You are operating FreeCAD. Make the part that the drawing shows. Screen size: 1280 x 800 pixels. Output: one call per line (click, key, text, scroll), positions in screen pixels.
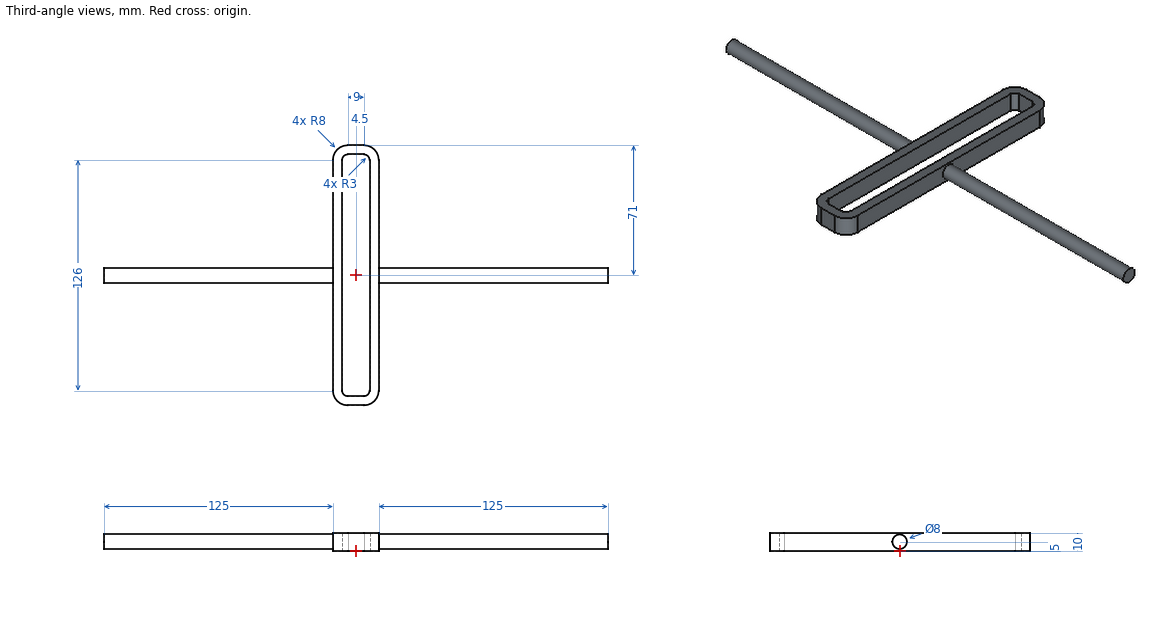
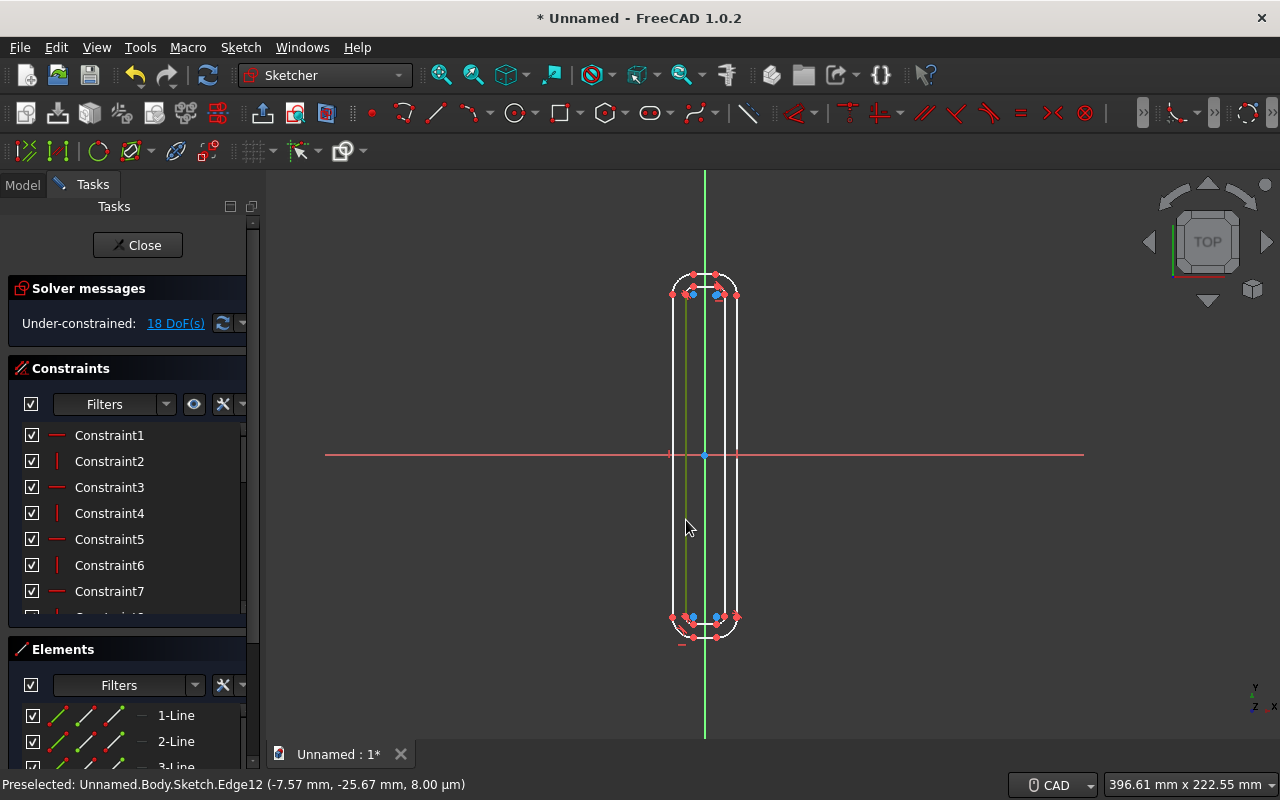
scroll(688, 622, up, 5)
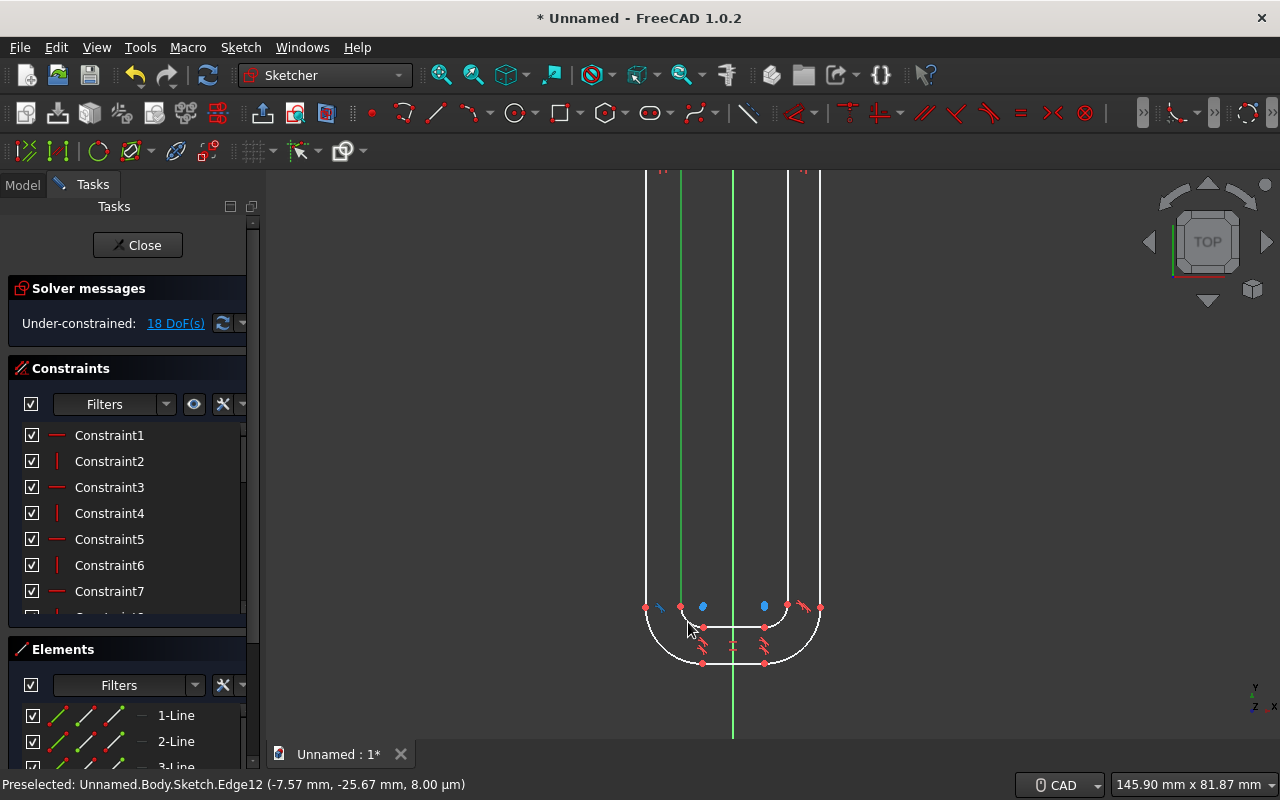
click(688, 621)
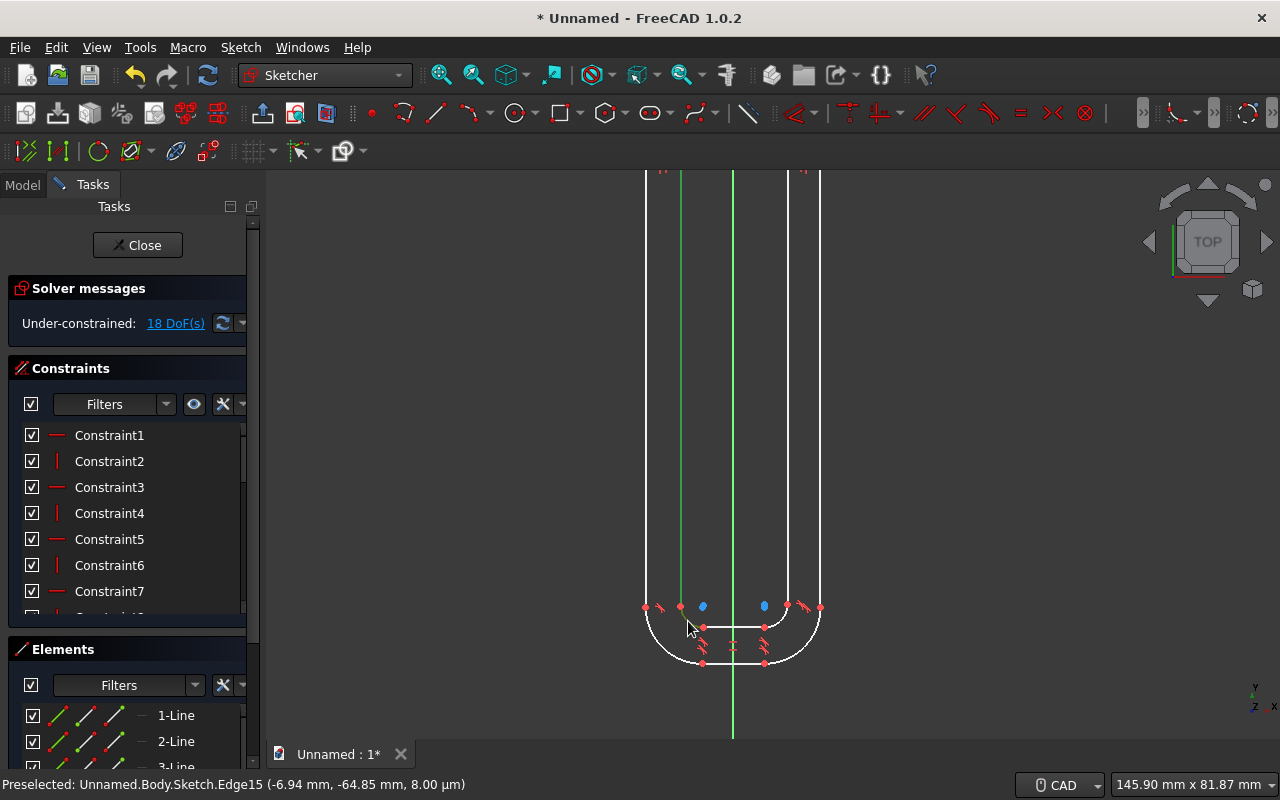
click(990, 114)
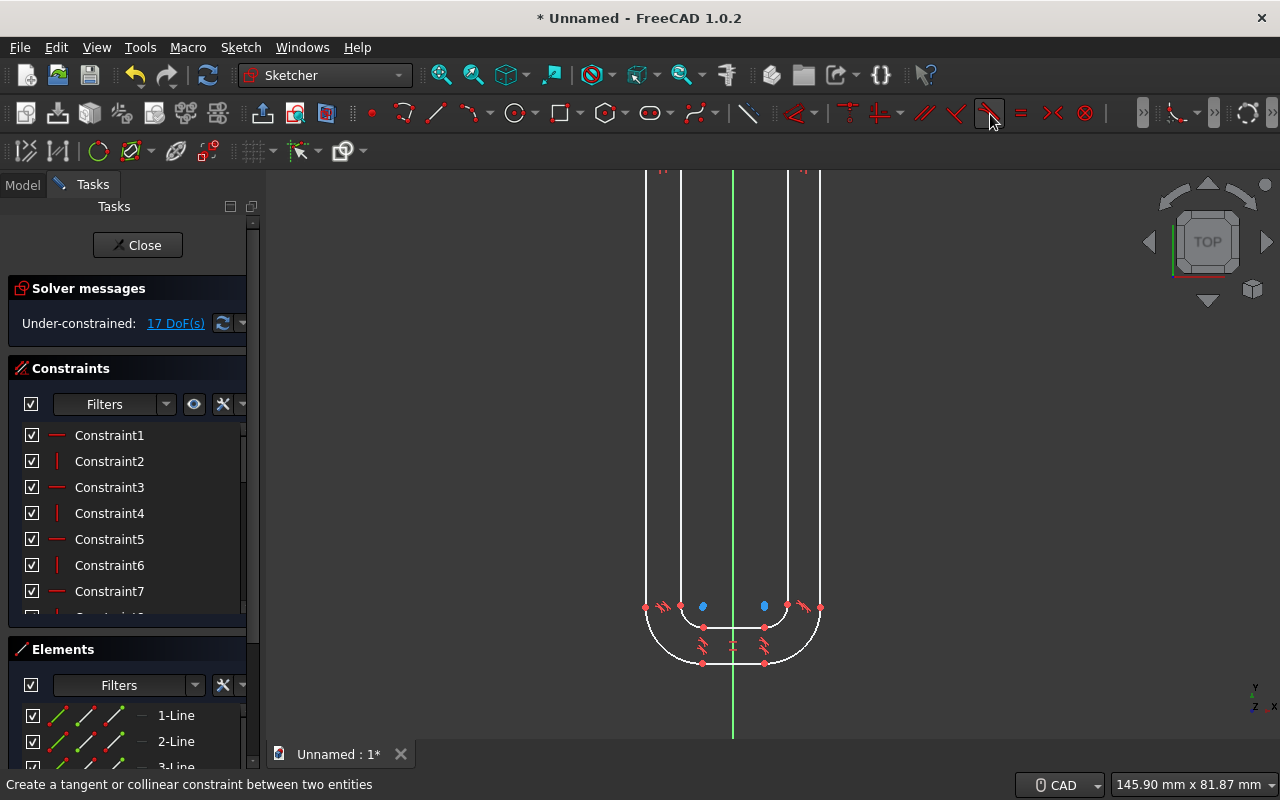
click(681, 343)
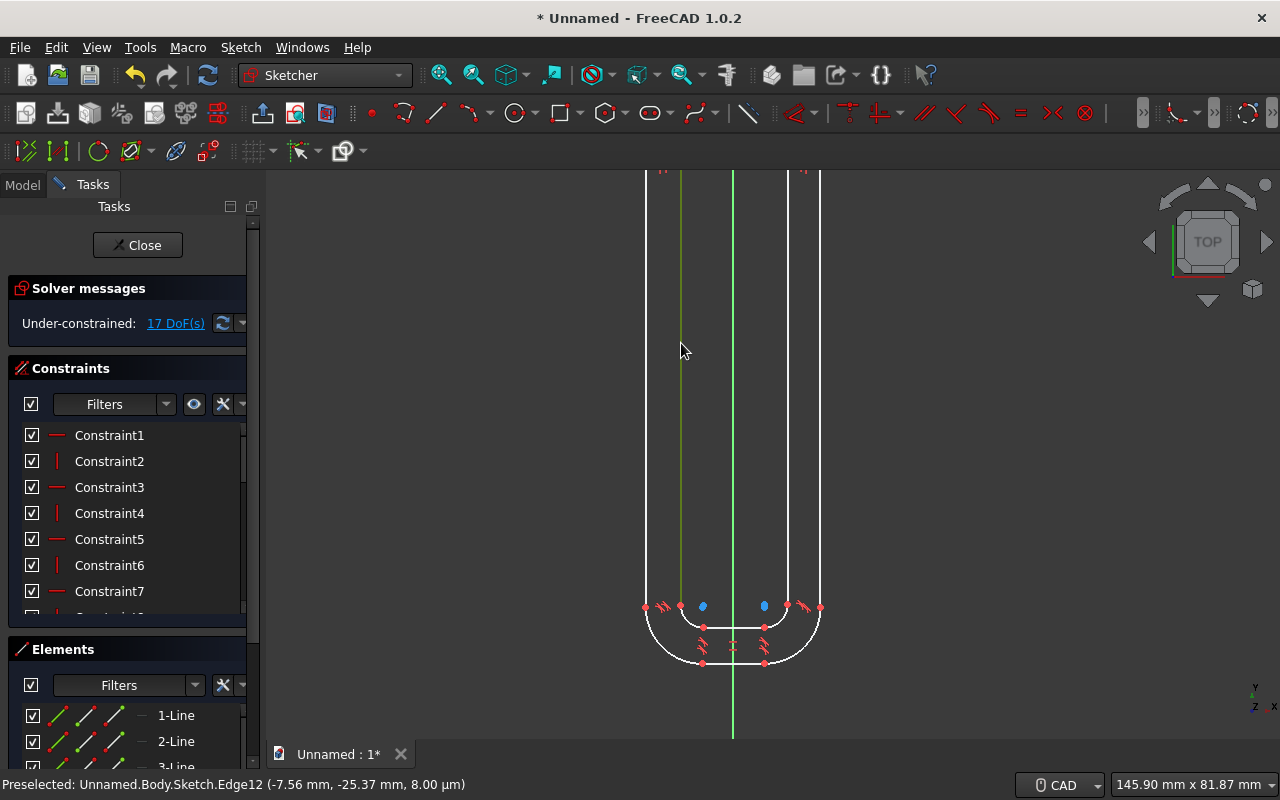
scroll(688, 621, down, 5)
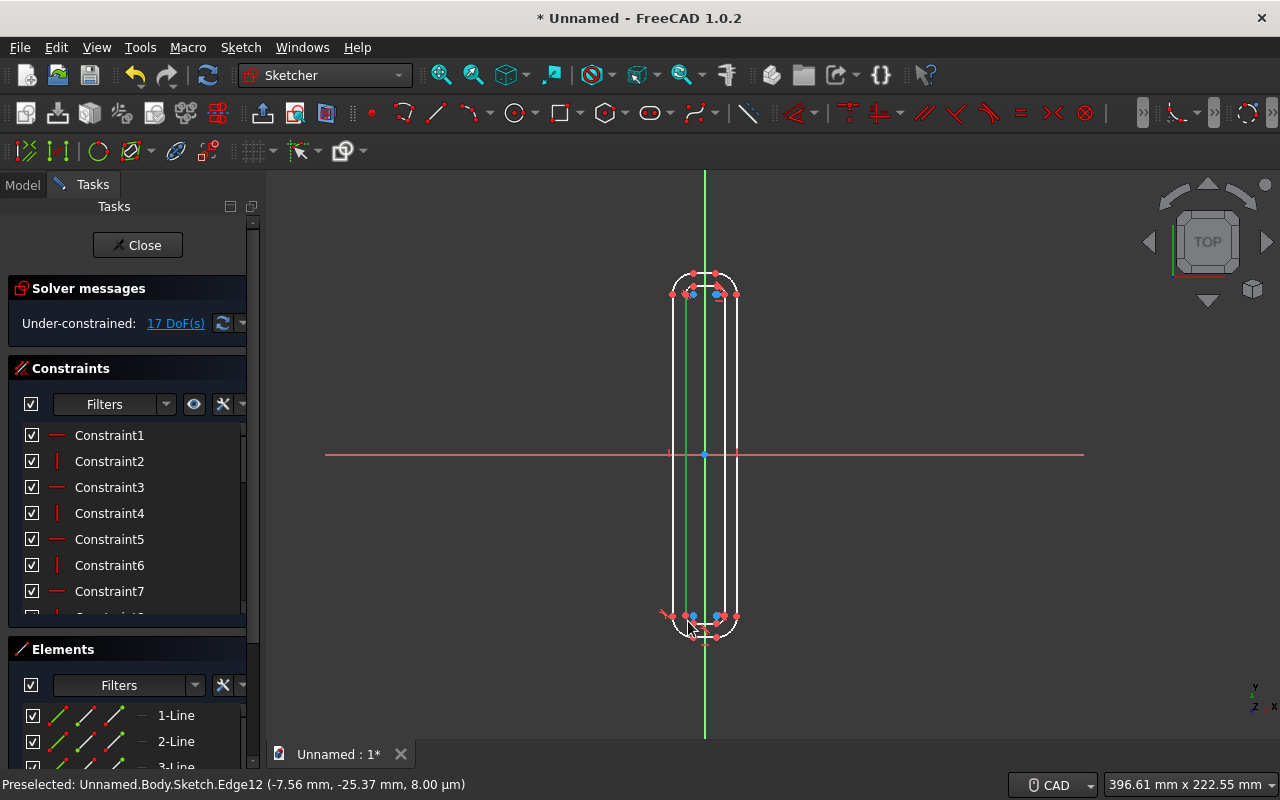
scroll(690, 287, up, 7)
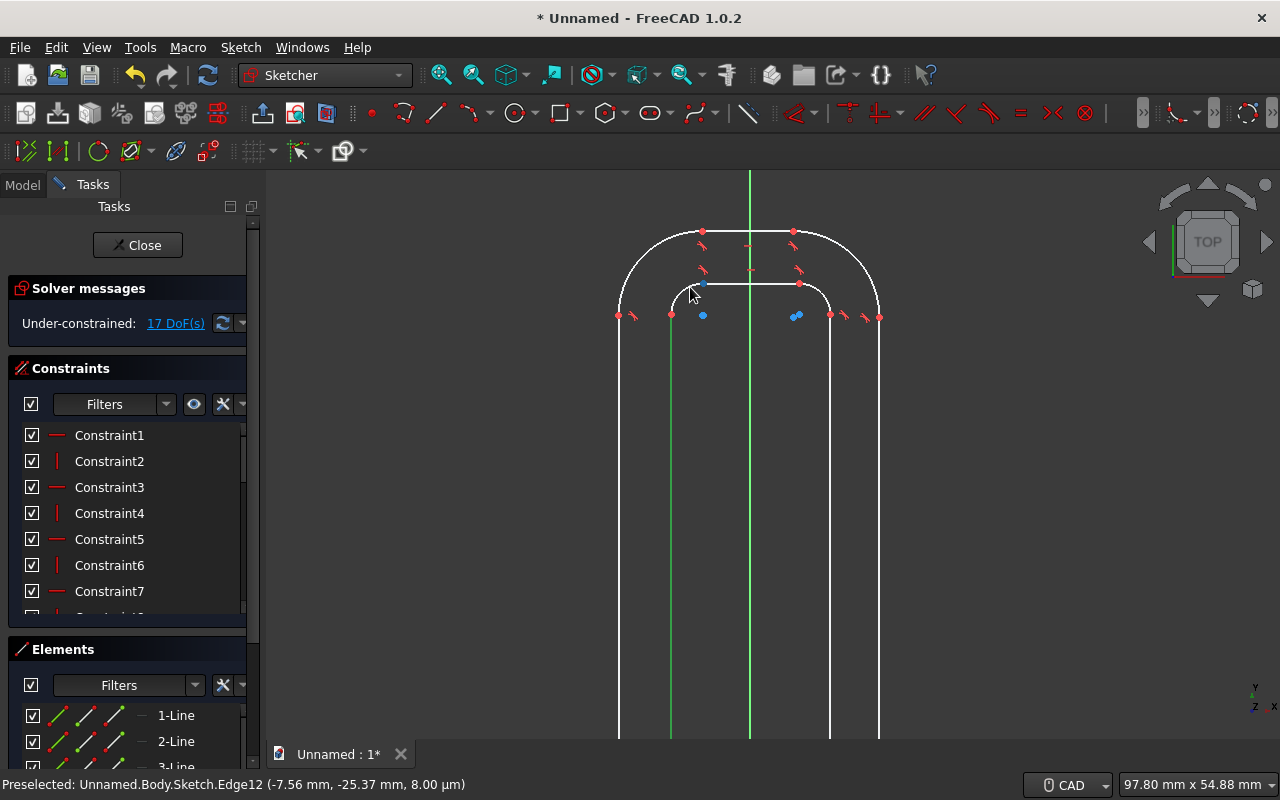
click(689, 287)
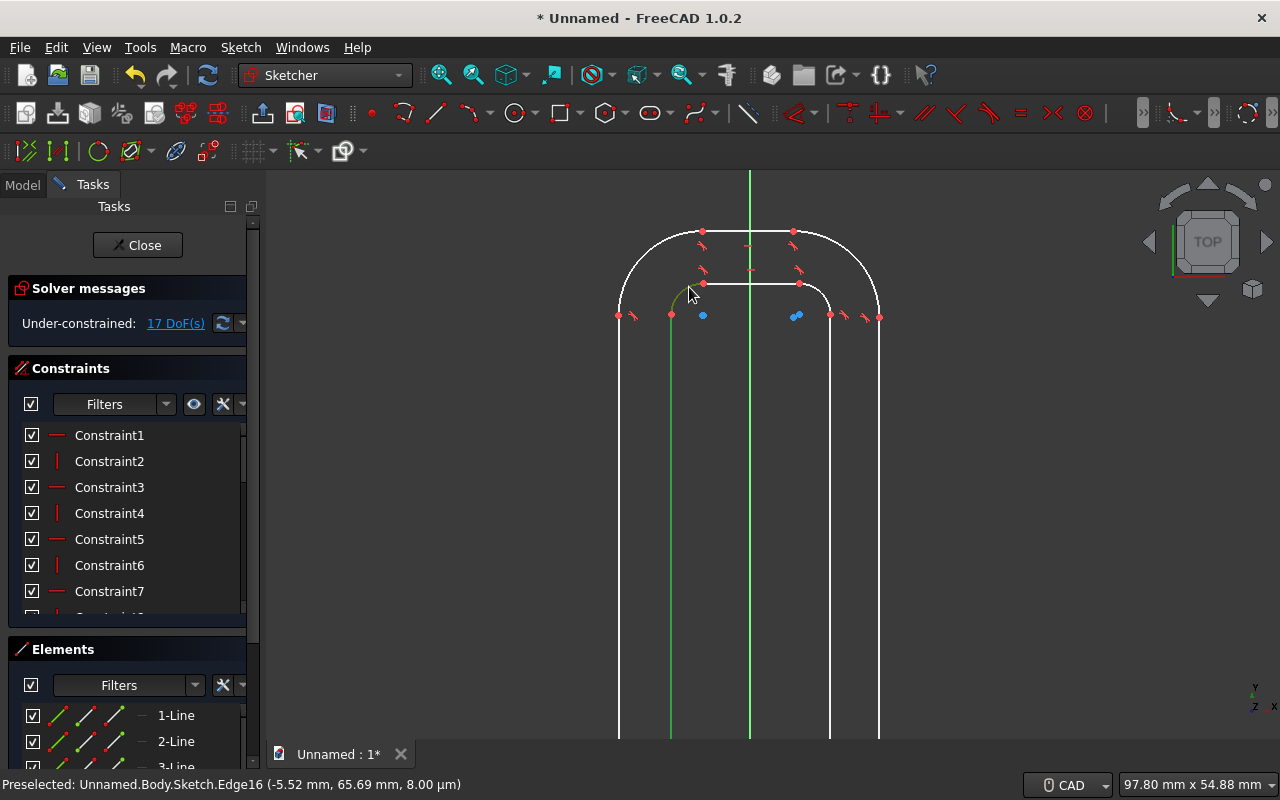
click(990, 114)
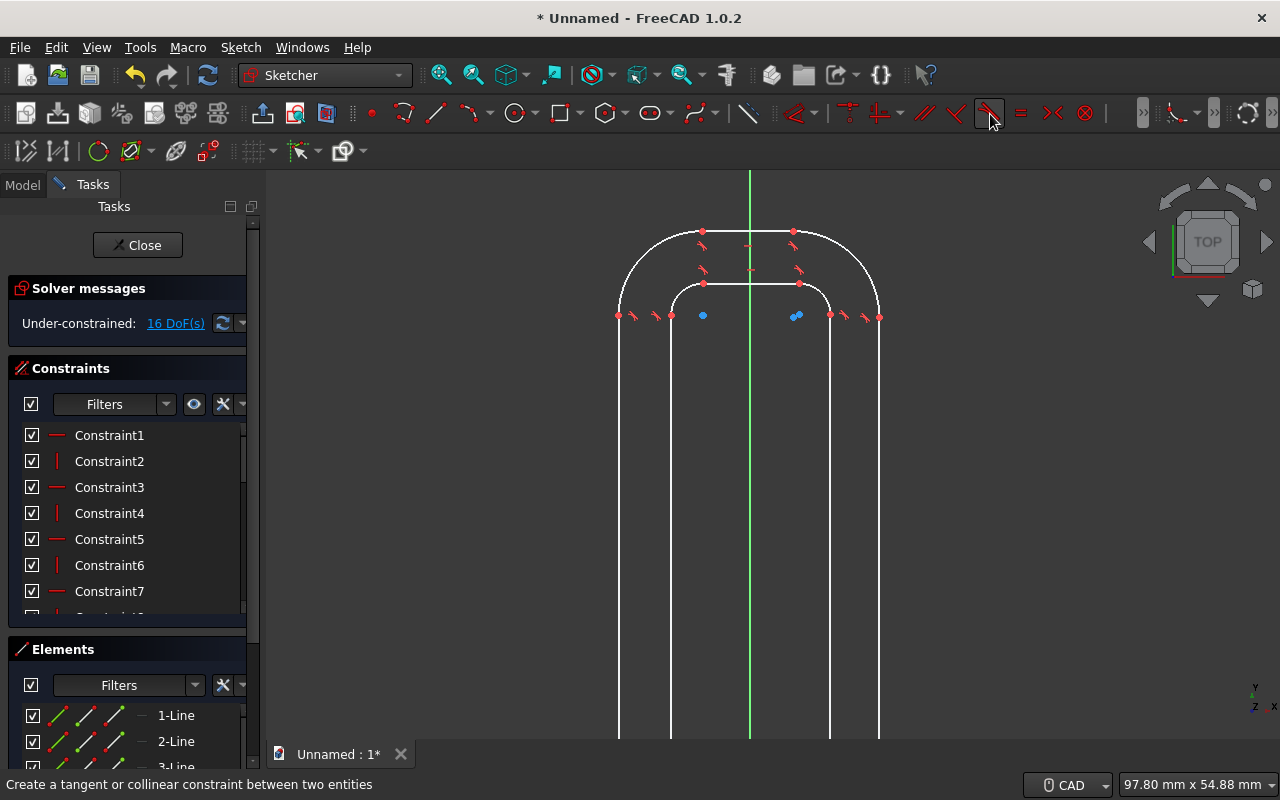
scroll(690, 287, down, 7)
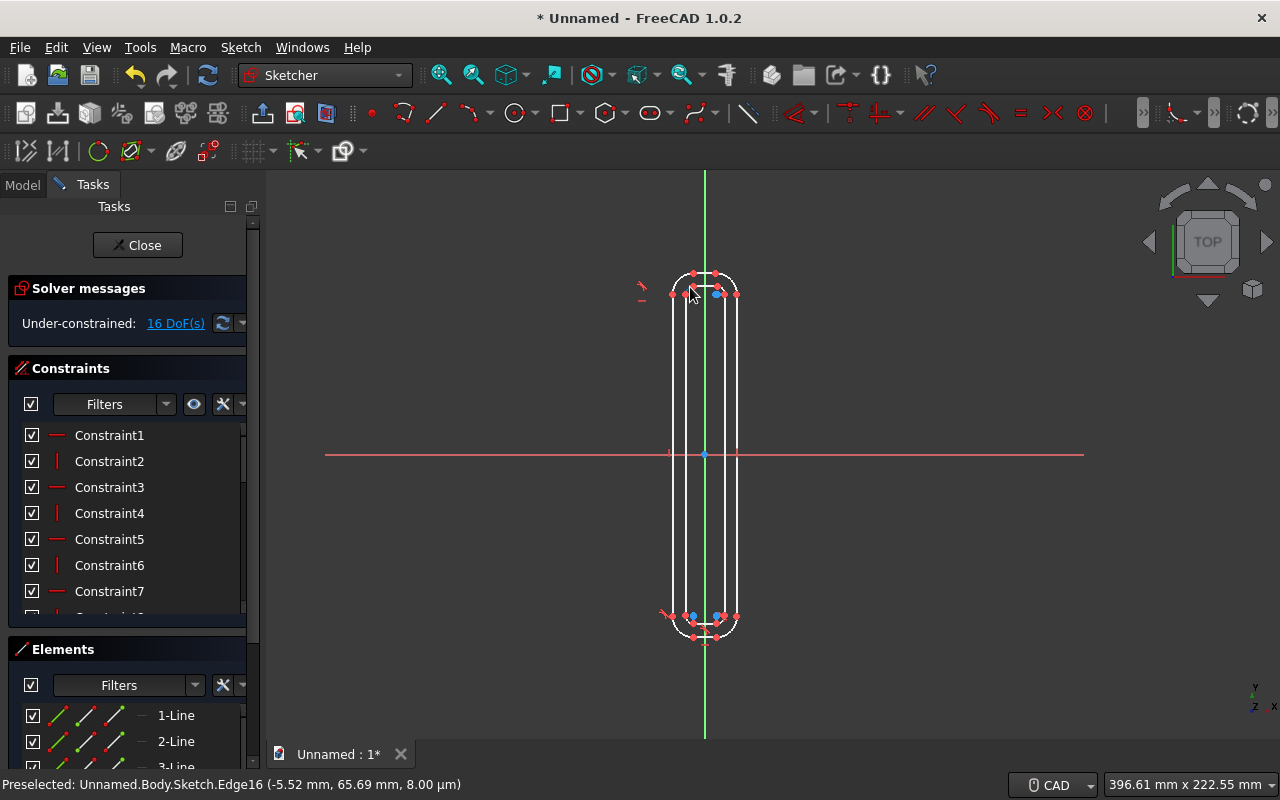
scroll(735, 285, up, 2)